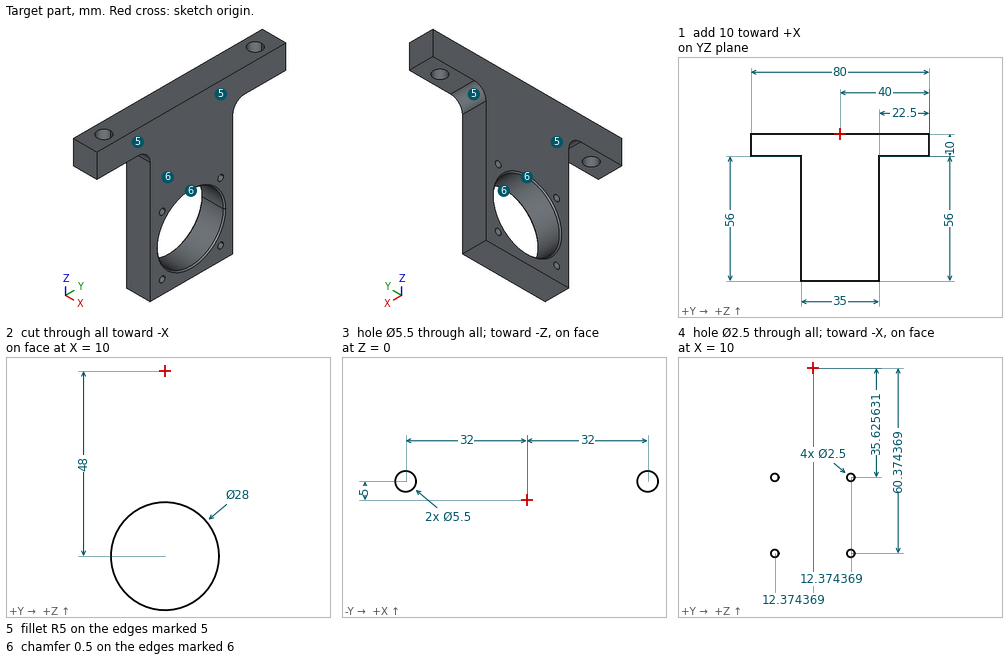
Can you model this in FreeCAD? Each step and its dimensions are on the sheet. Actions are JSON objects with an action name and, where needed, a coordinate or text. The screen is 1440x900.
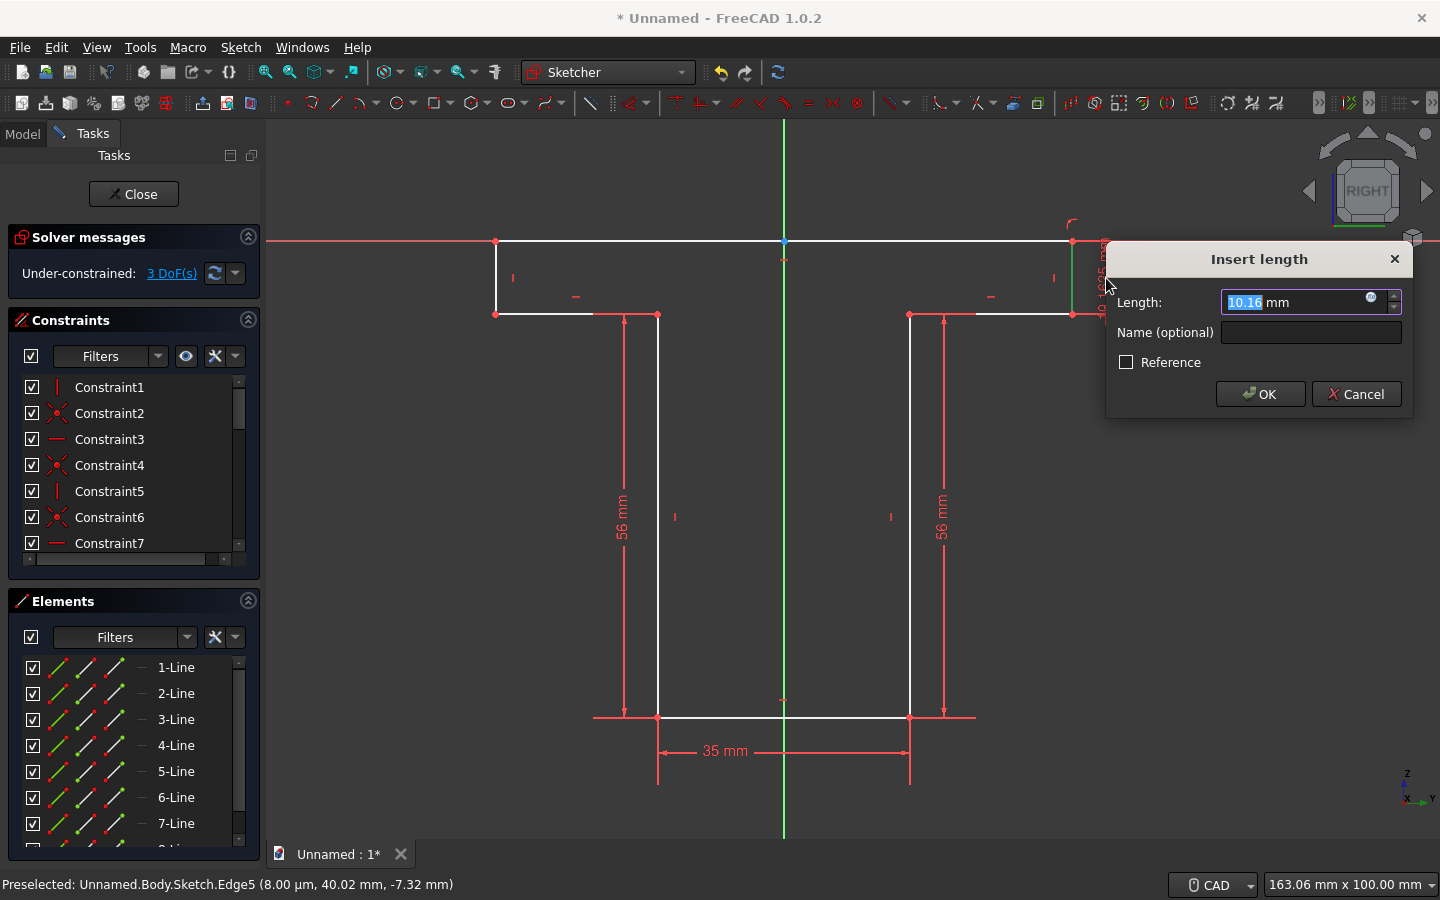
{"action": "type", "text": "10"}
{"action": "key", "text": "Return"}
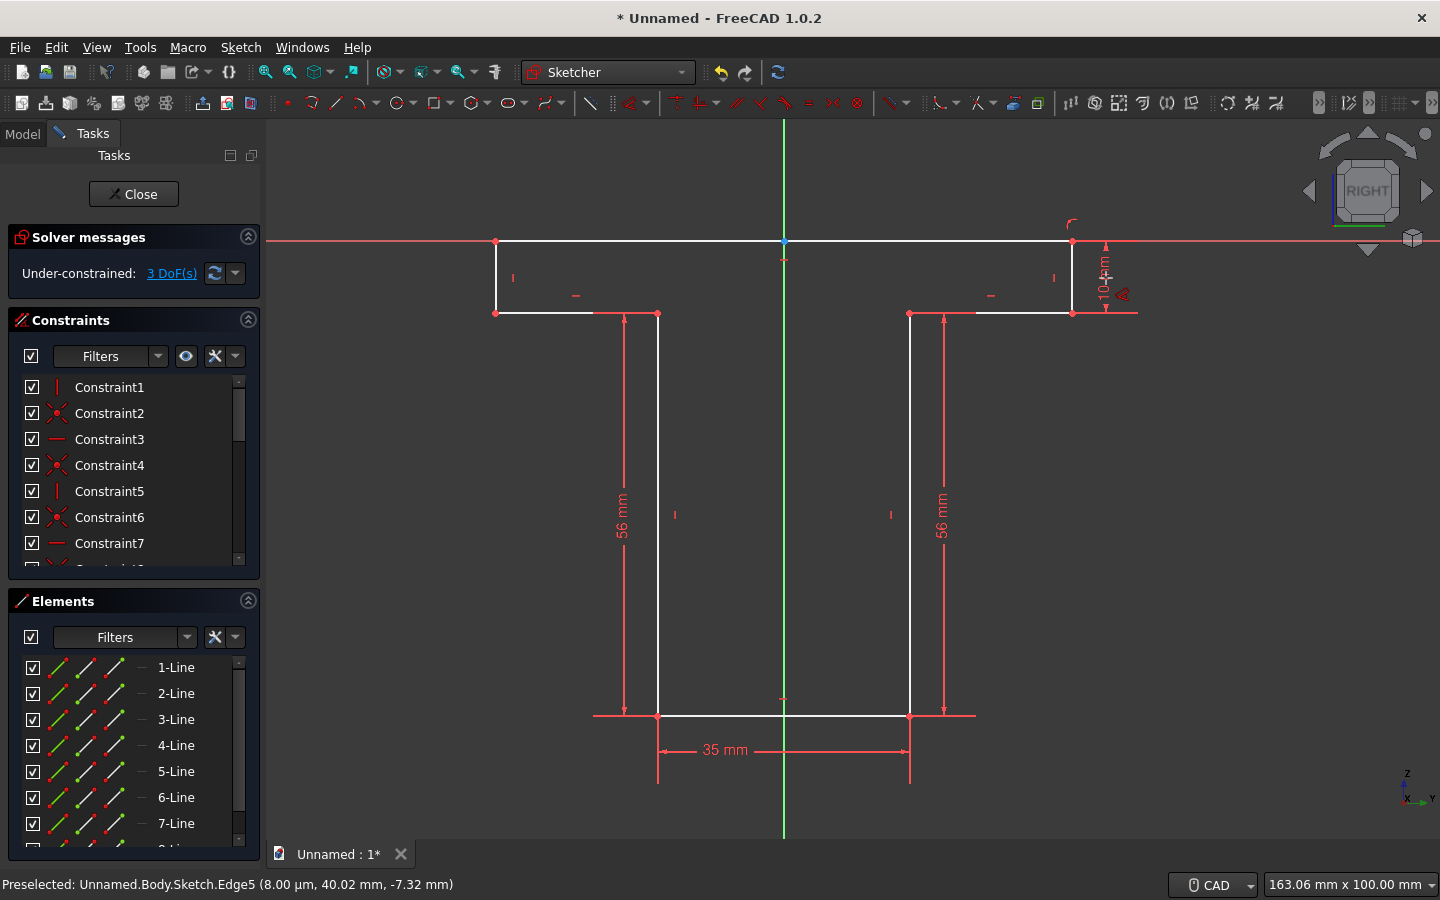
{"action": "left_click", "coordinate": [899, 241]}
{"action": "left_click", "coordinate": [652, 207]}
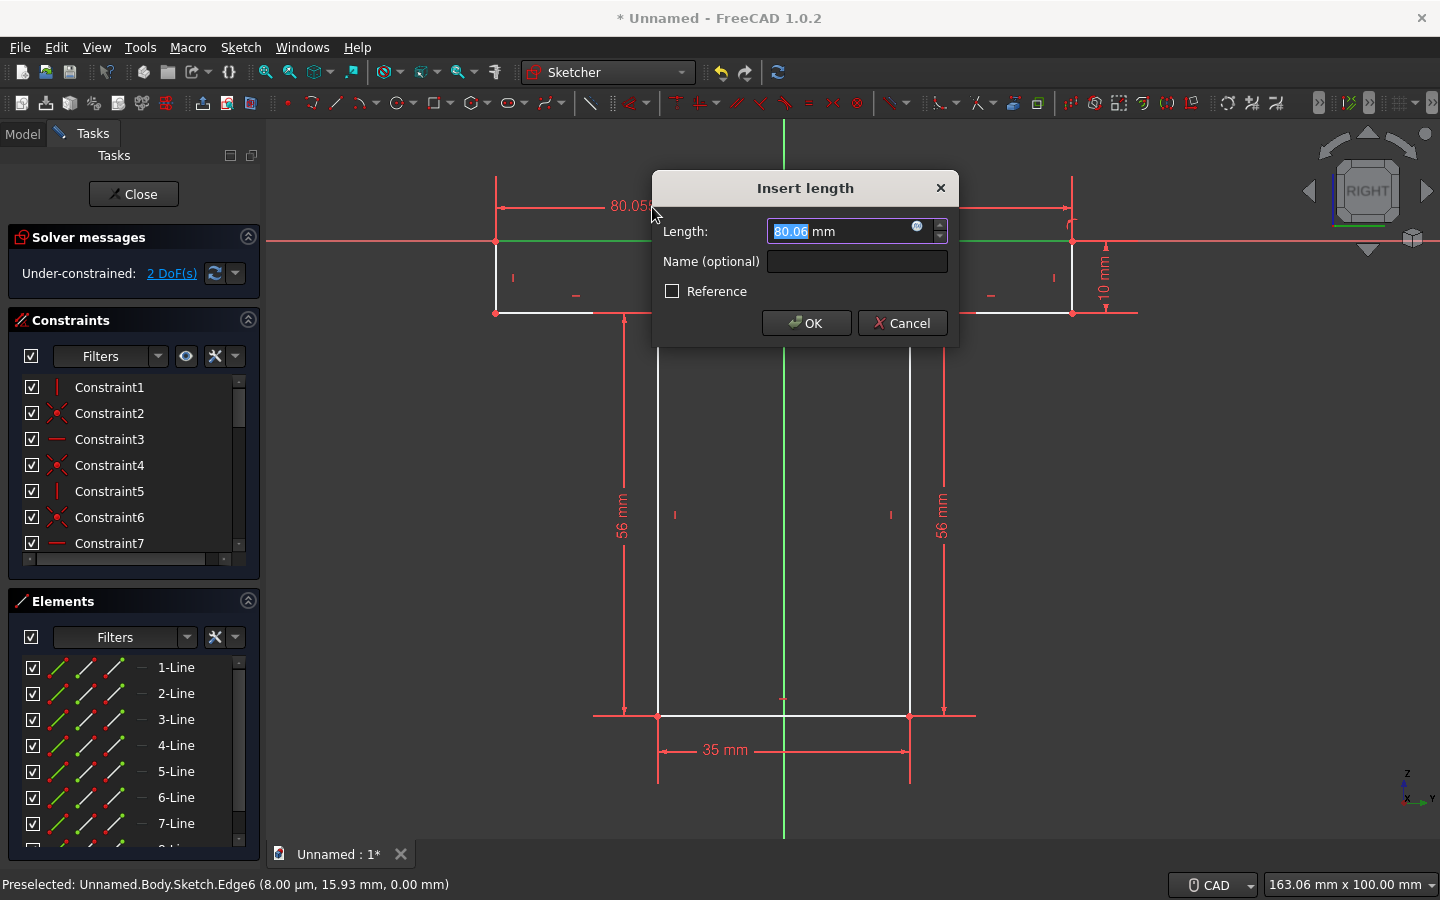
{"action": "type", "text": "80"}
{"action": "key", "text": "Return"}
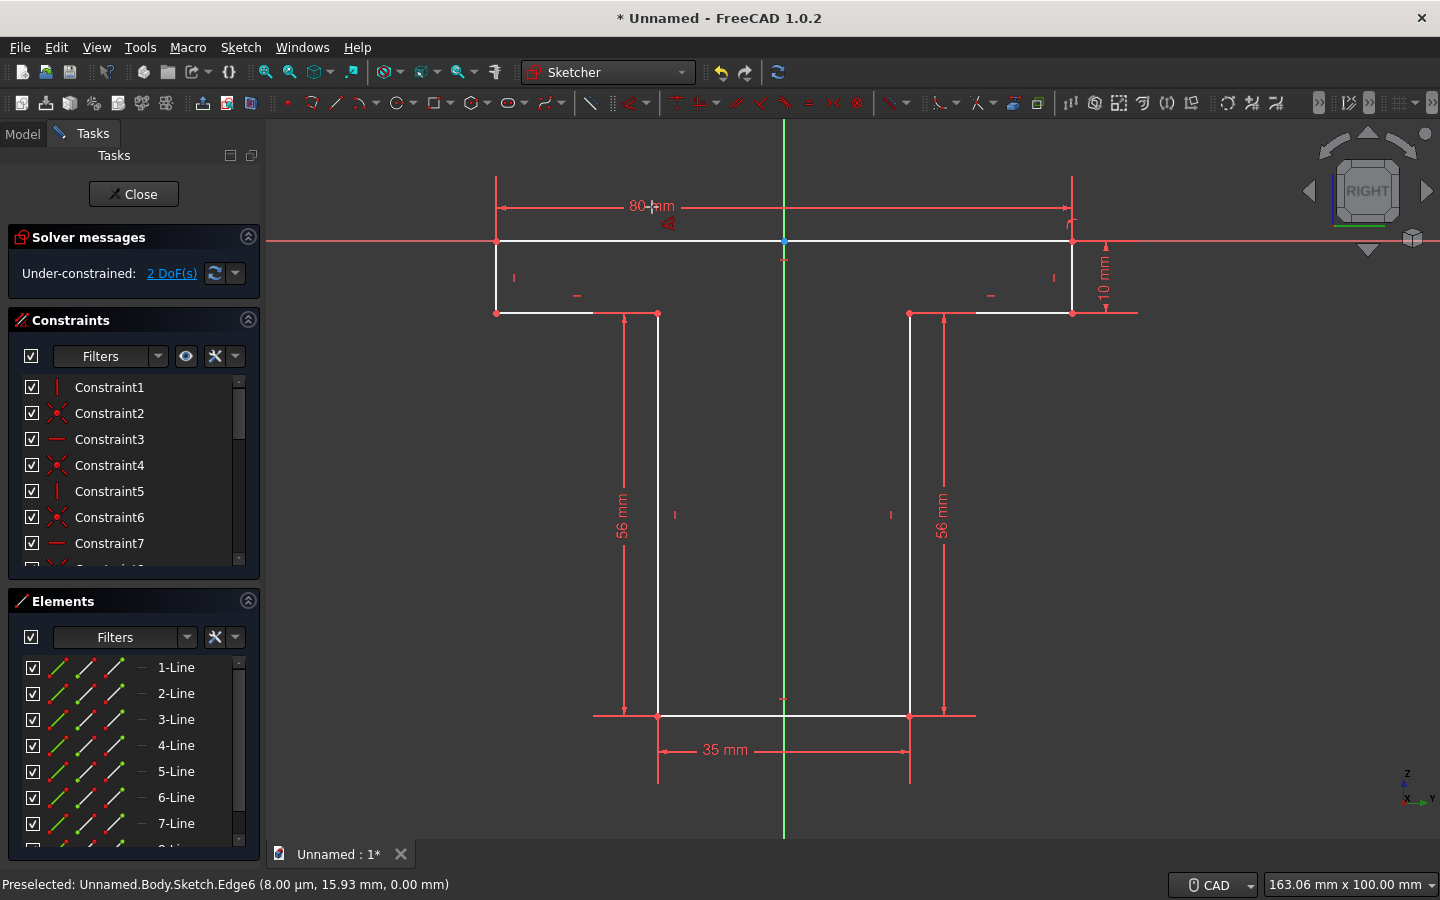
{"action": "left_click", "coordinate": [1072, 313]}
{"action": "left_click", "coordinate": [928, 207]}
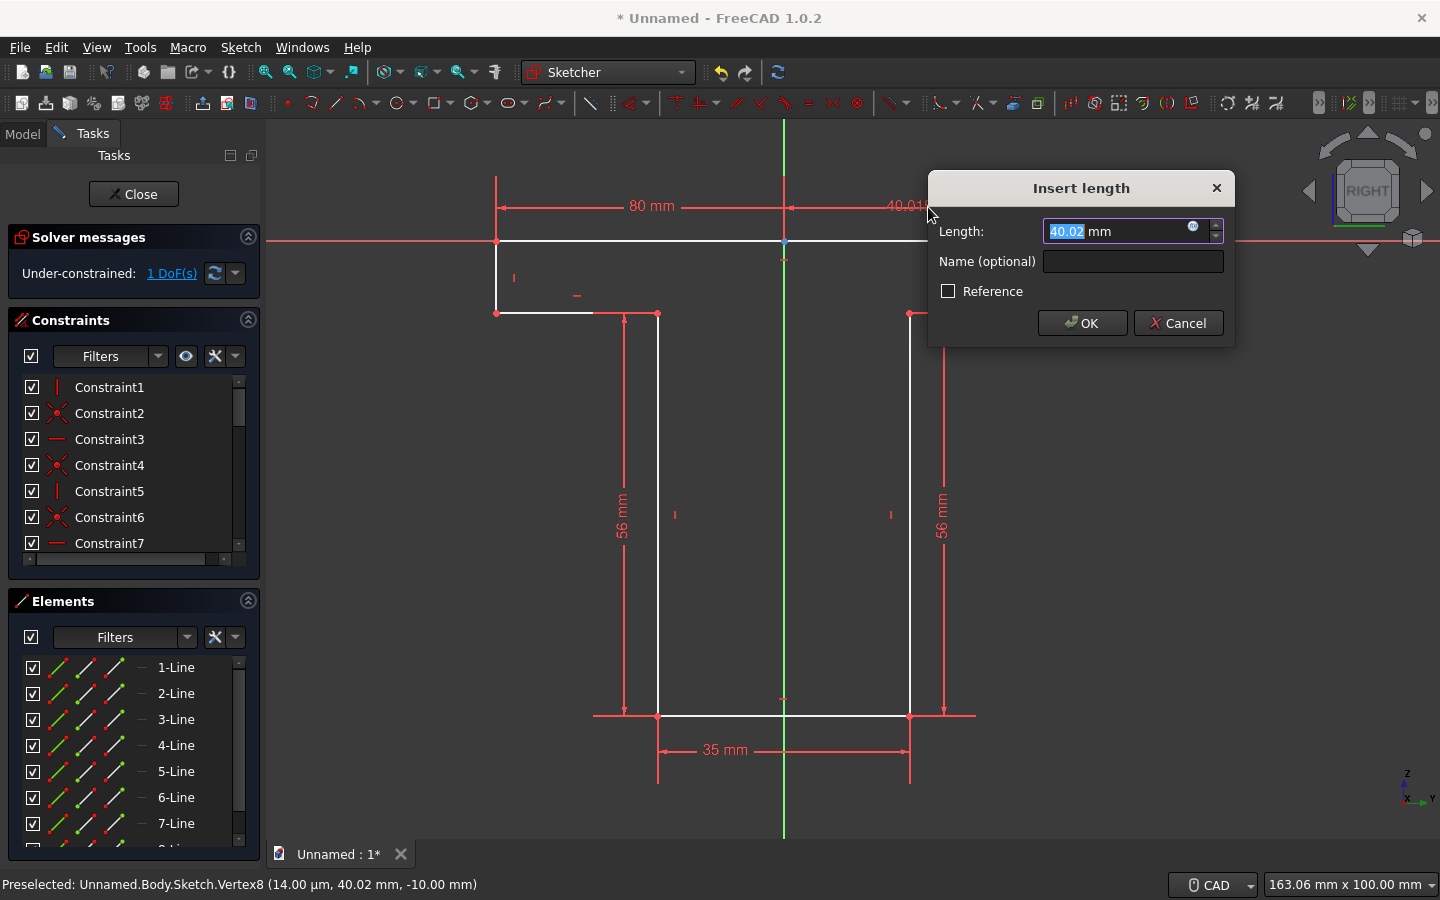
{"action": "type", "text": "40"}
{"action": "key", "text": "Return"}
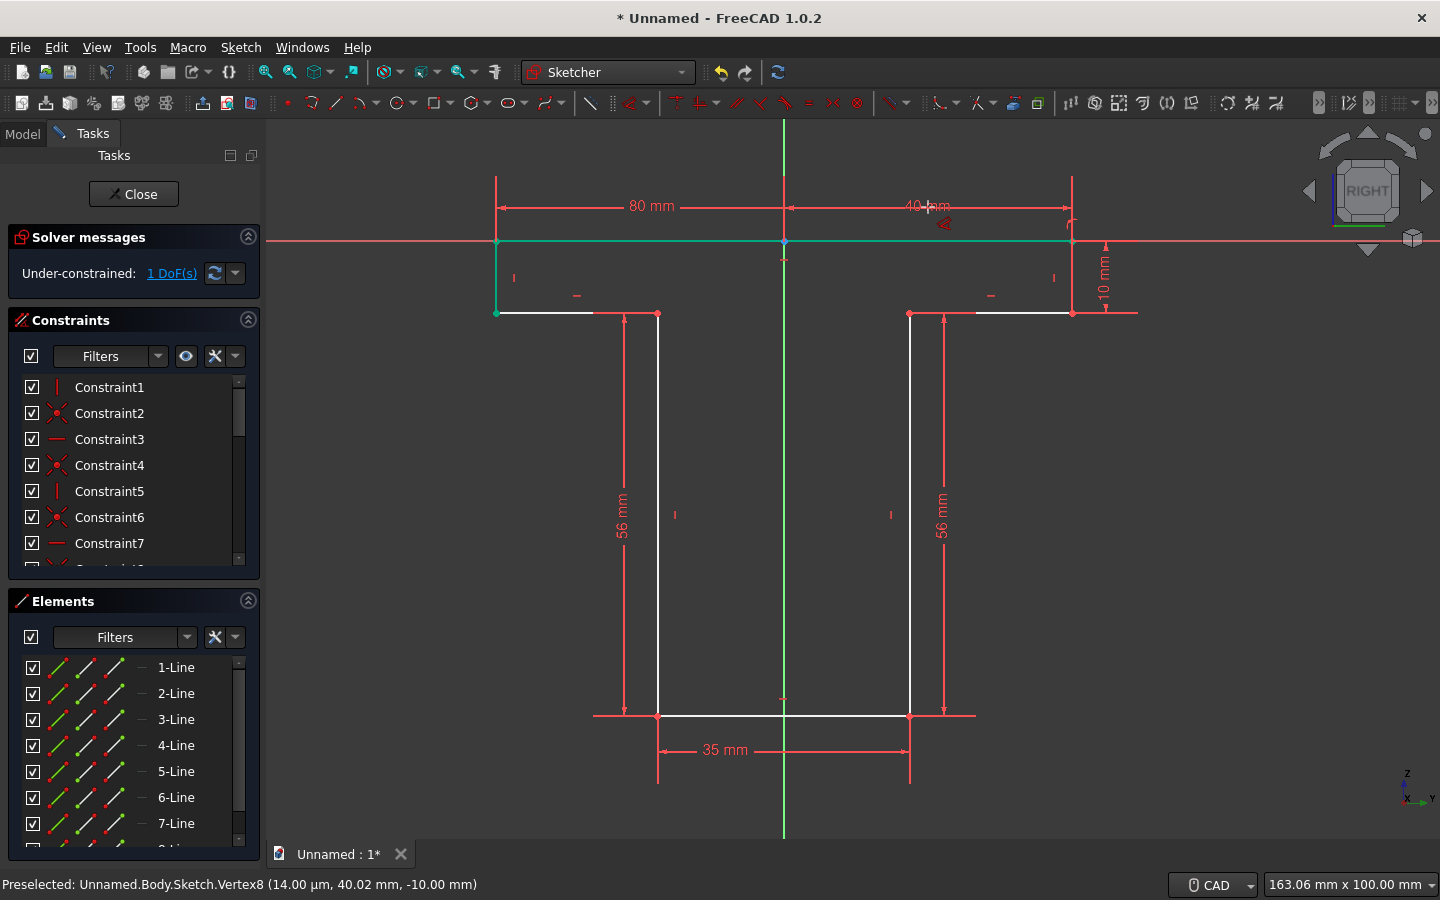
{"action": "left_click", "coordinate": [959, 313]}
{"action": "left_click", "coordinate": [991, 279]}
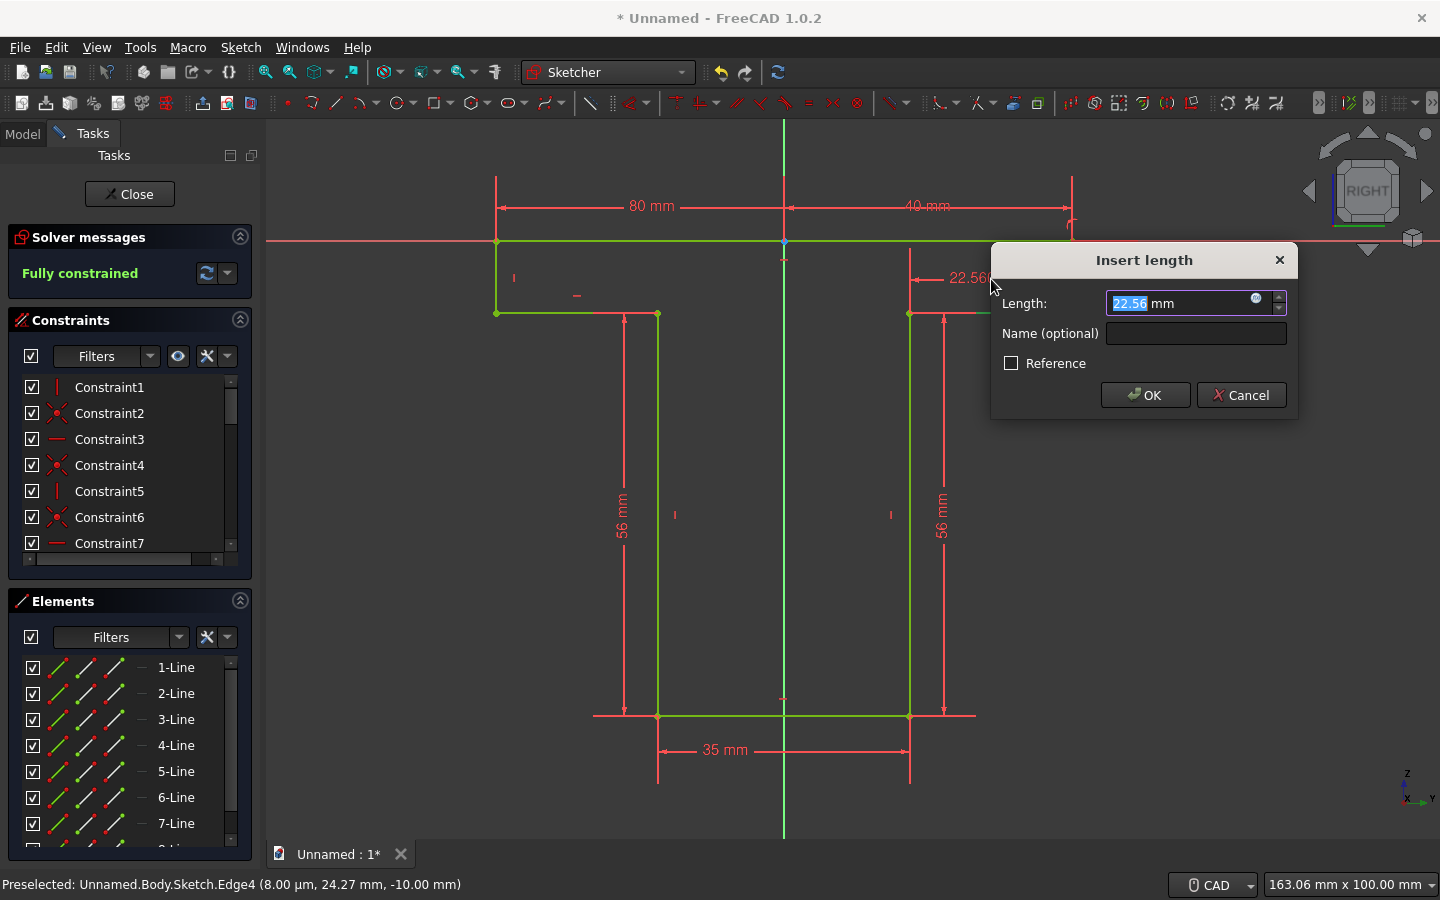
{"action": "type", "text": "22.5"}
{"action": "key", "text": "Return"}
{"action": "key", "text": "Escape"}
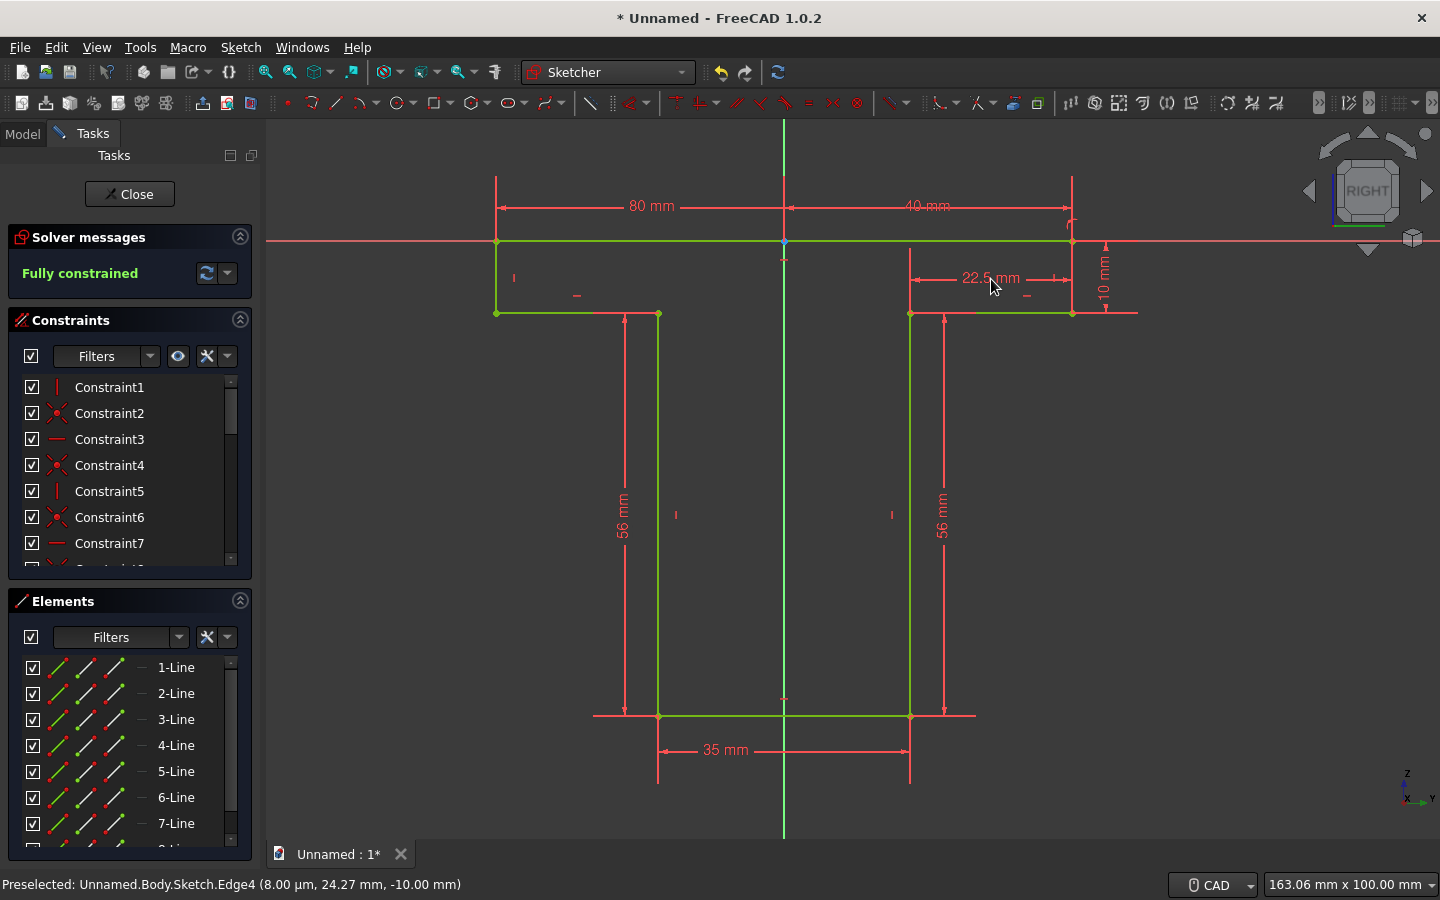
{"action": "left_click", "coordinate": [130, 194]}